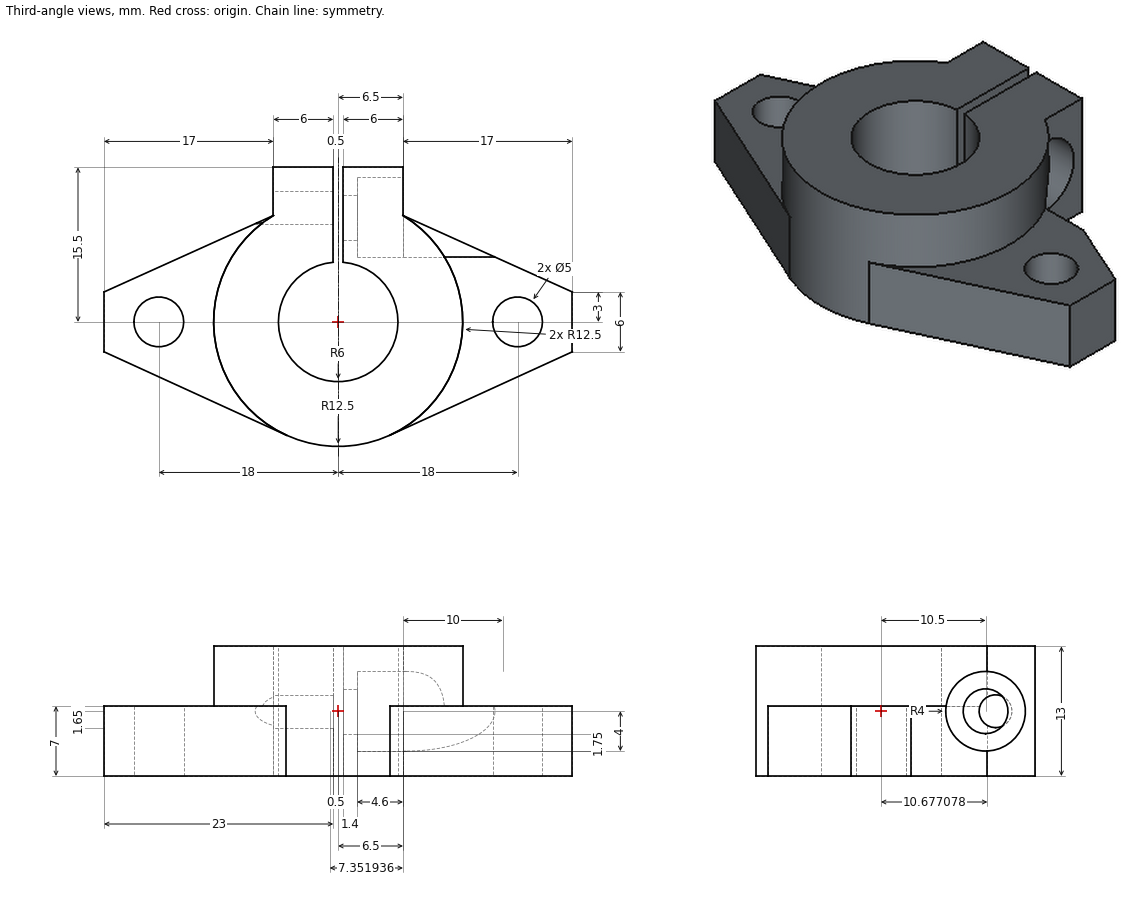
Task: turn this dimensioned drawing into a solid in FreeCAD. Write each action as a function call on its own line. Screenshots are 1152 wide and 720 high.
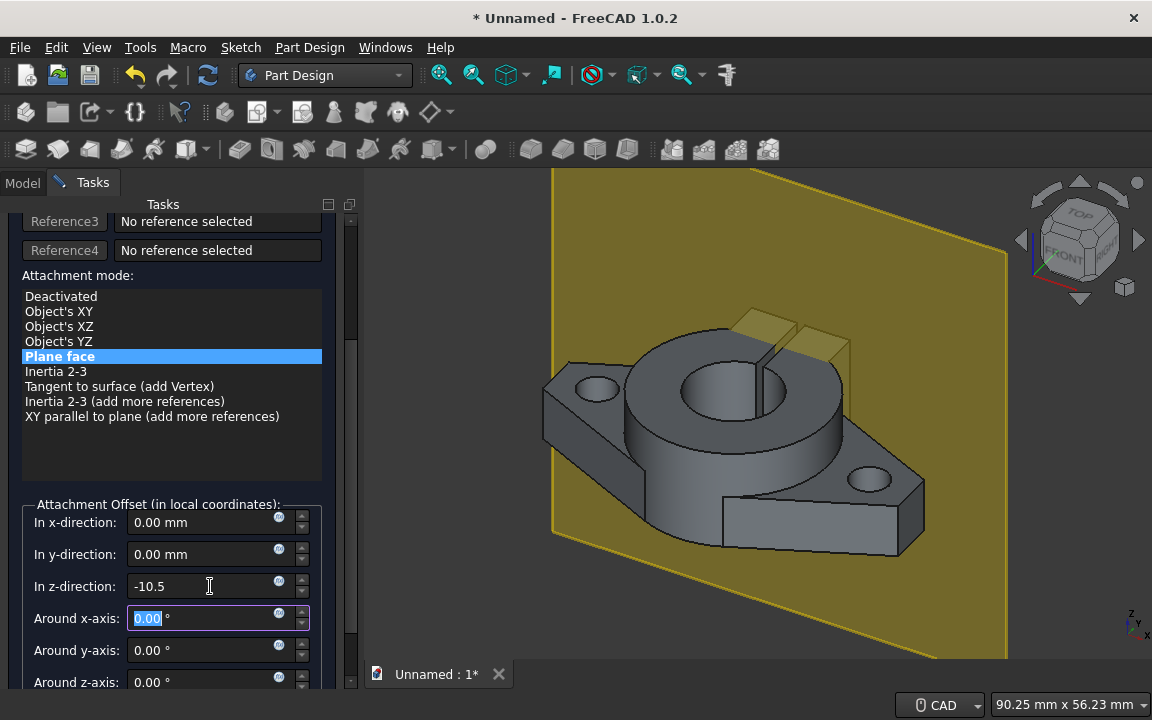
scroll(351, 451, up, 4)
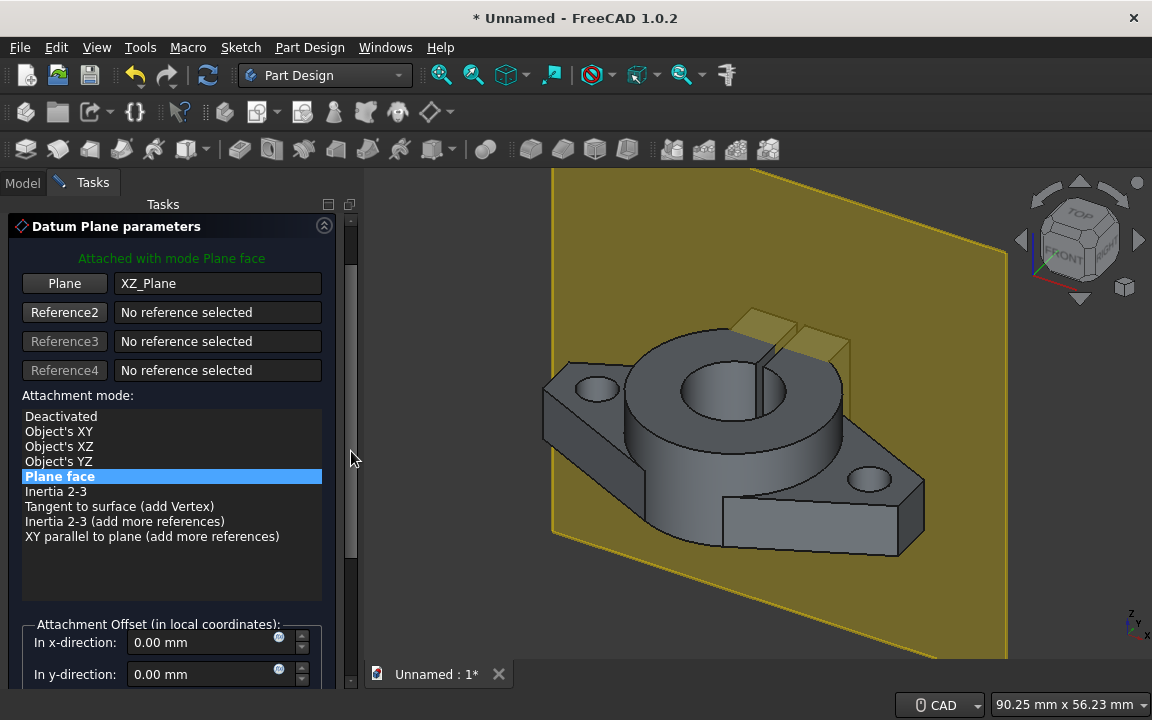
click(124, 243)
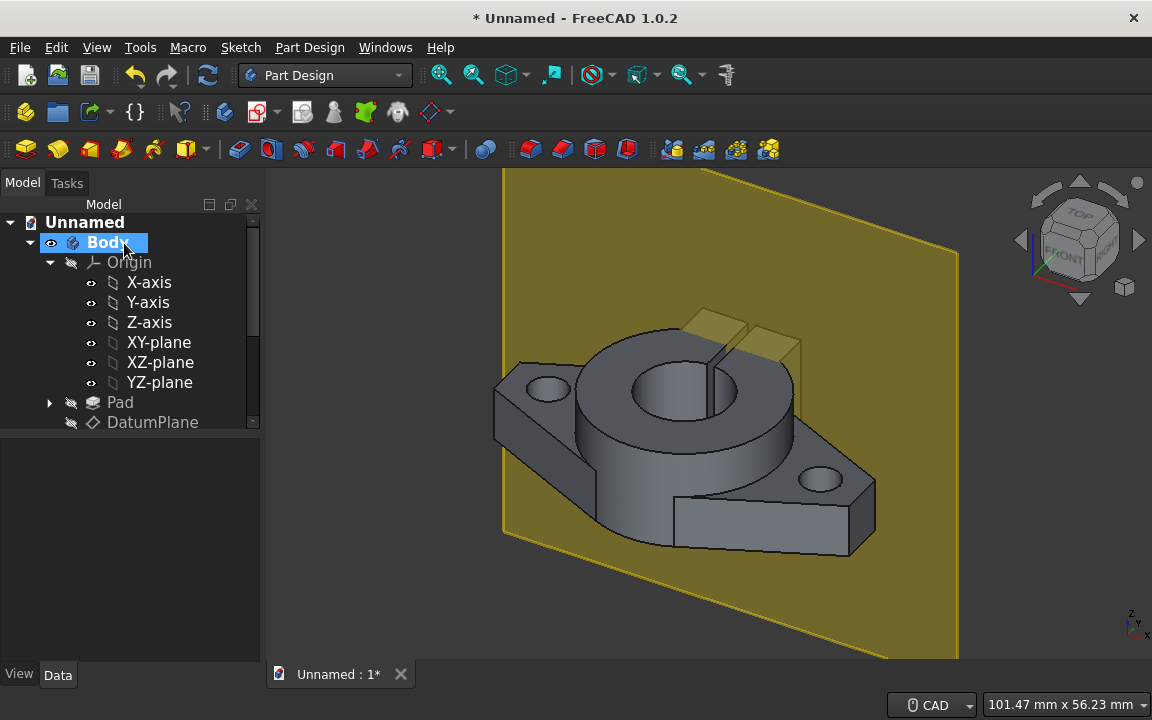
scroll(100, 318, down, 3)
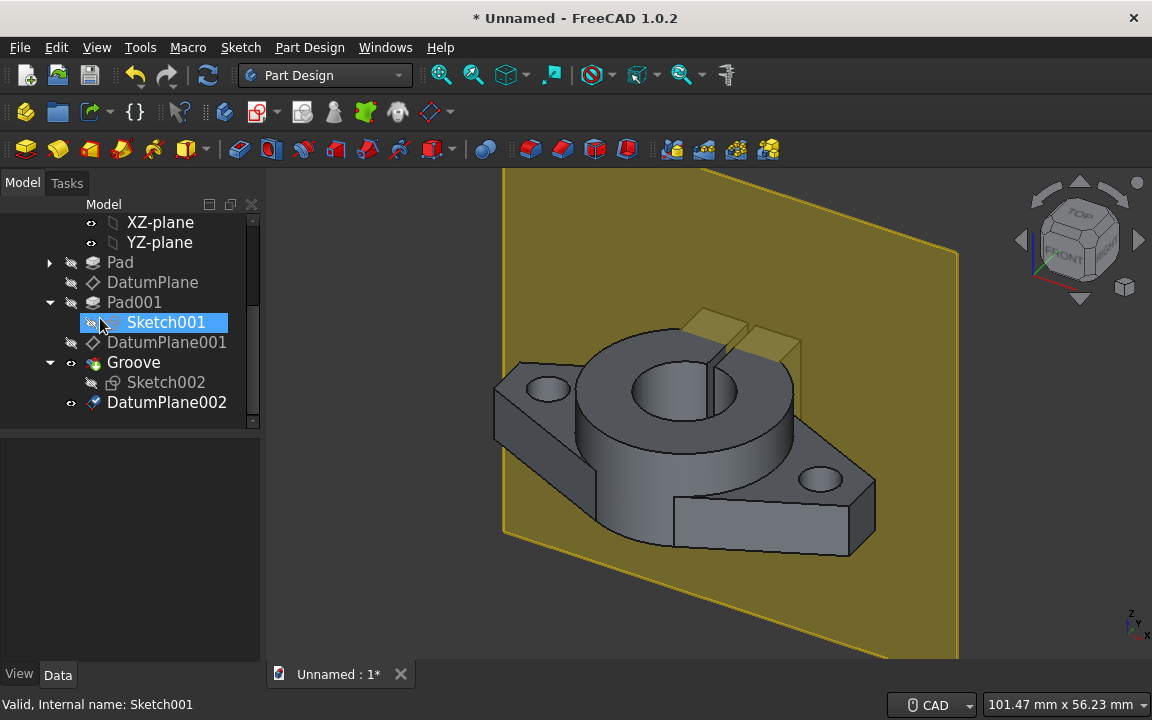
click(116, 403)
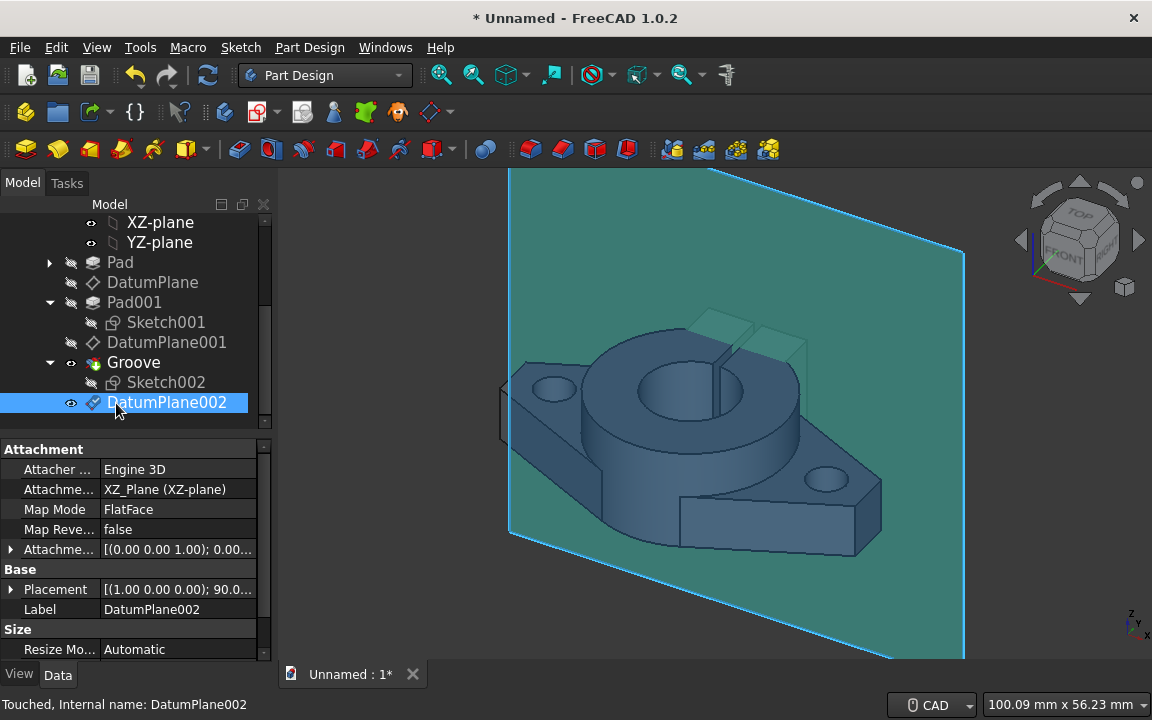
click(258, 112)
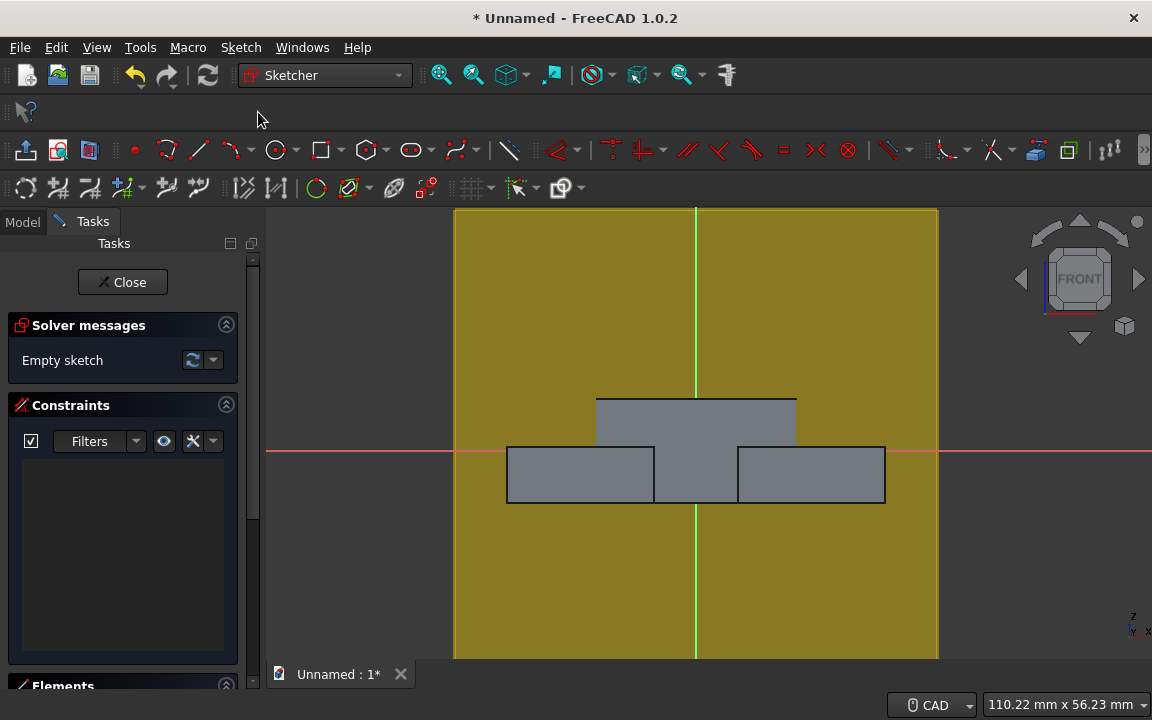
click(90, 150)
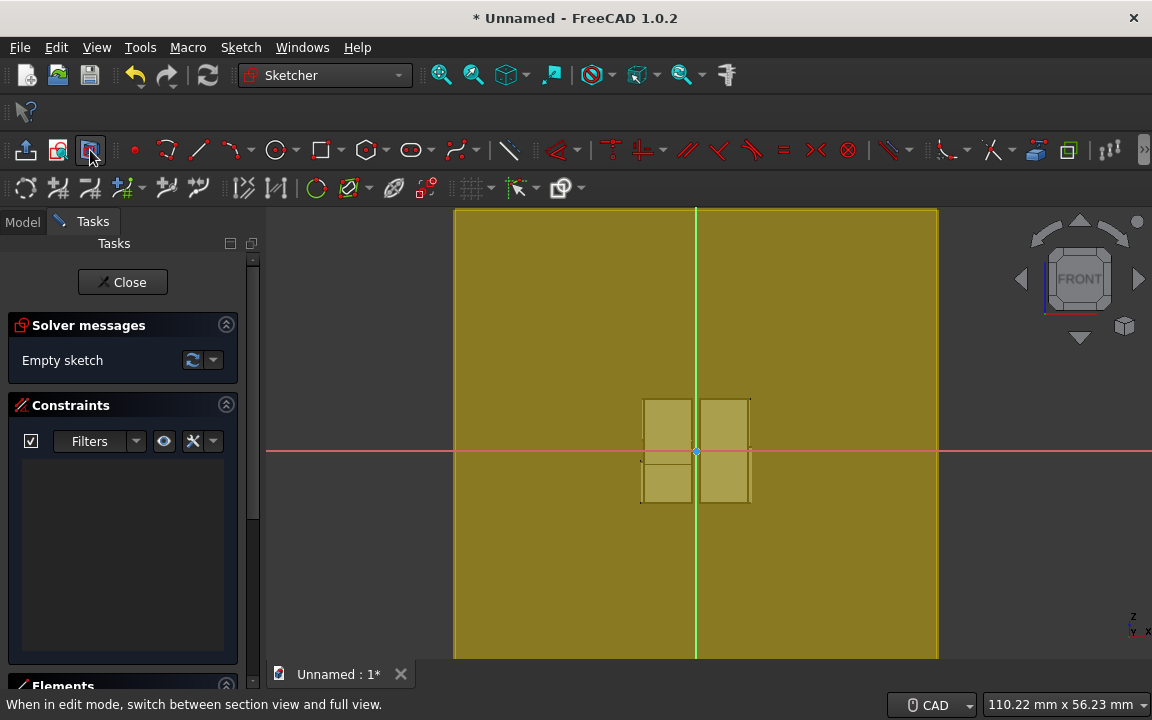
scroll(729, 471, up, 11)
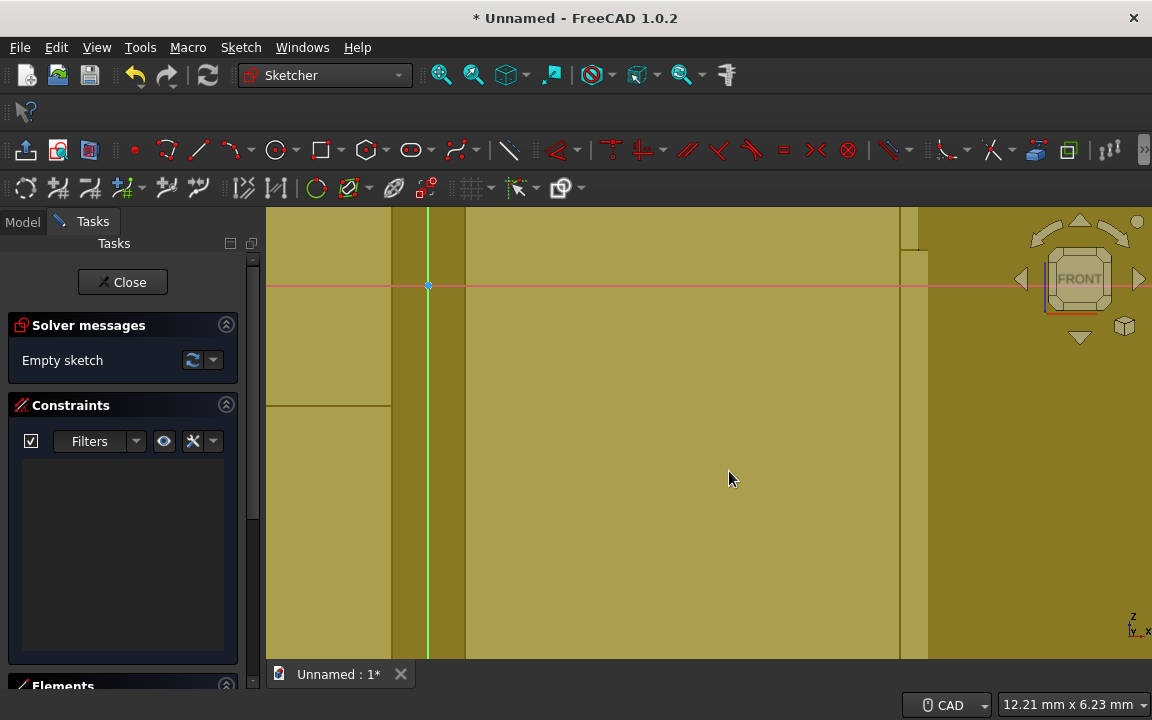
click(168, 150)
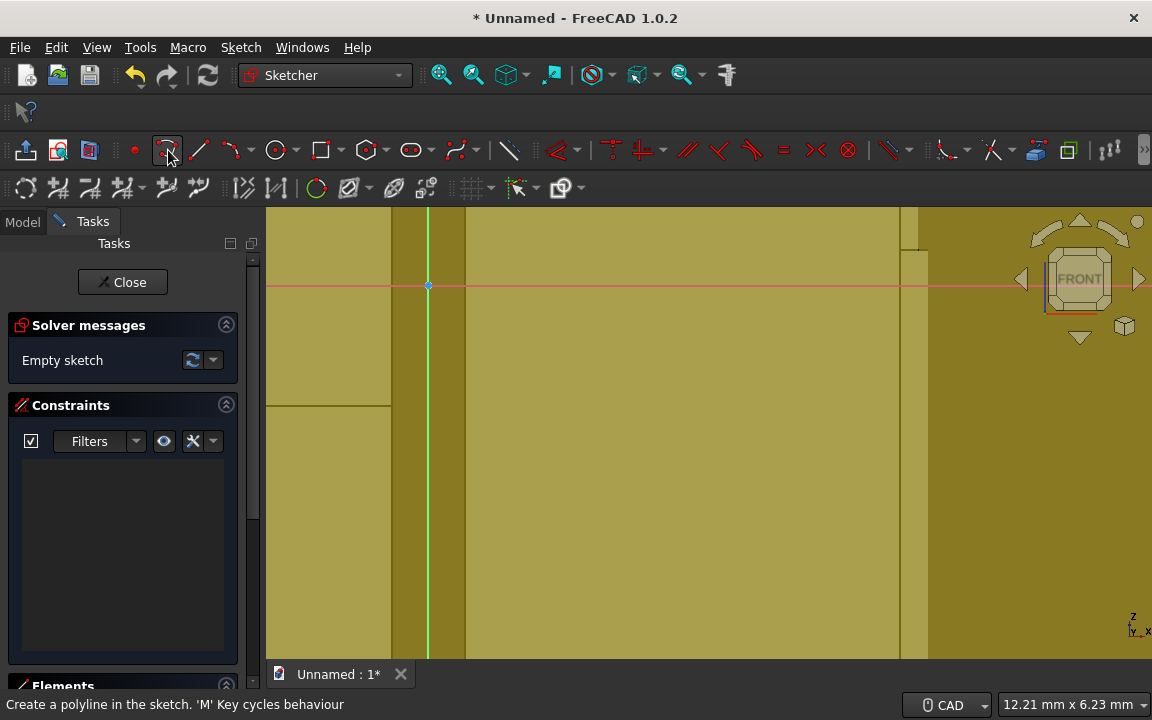
click(366, 286)
click(900, 295)
click(900, 576)
click(566, 576)
click(566, 449)
click(465, 449)
click(366, 286)
key(Escape)
key(Escape)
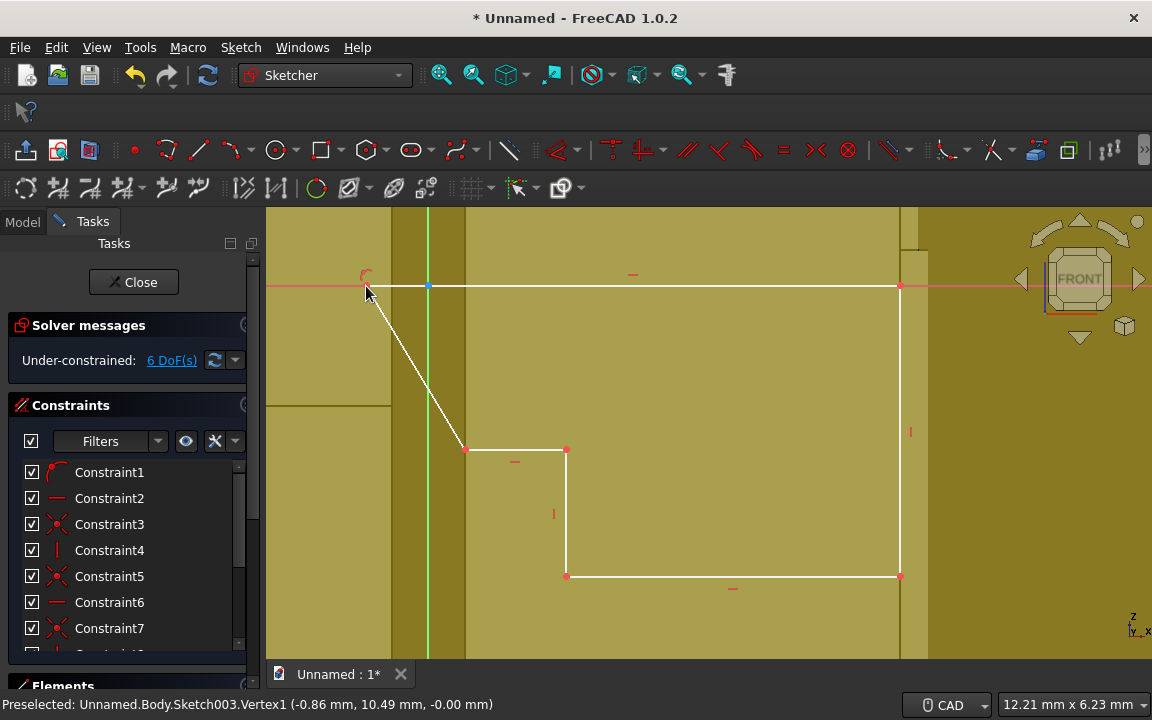
click(556, 150)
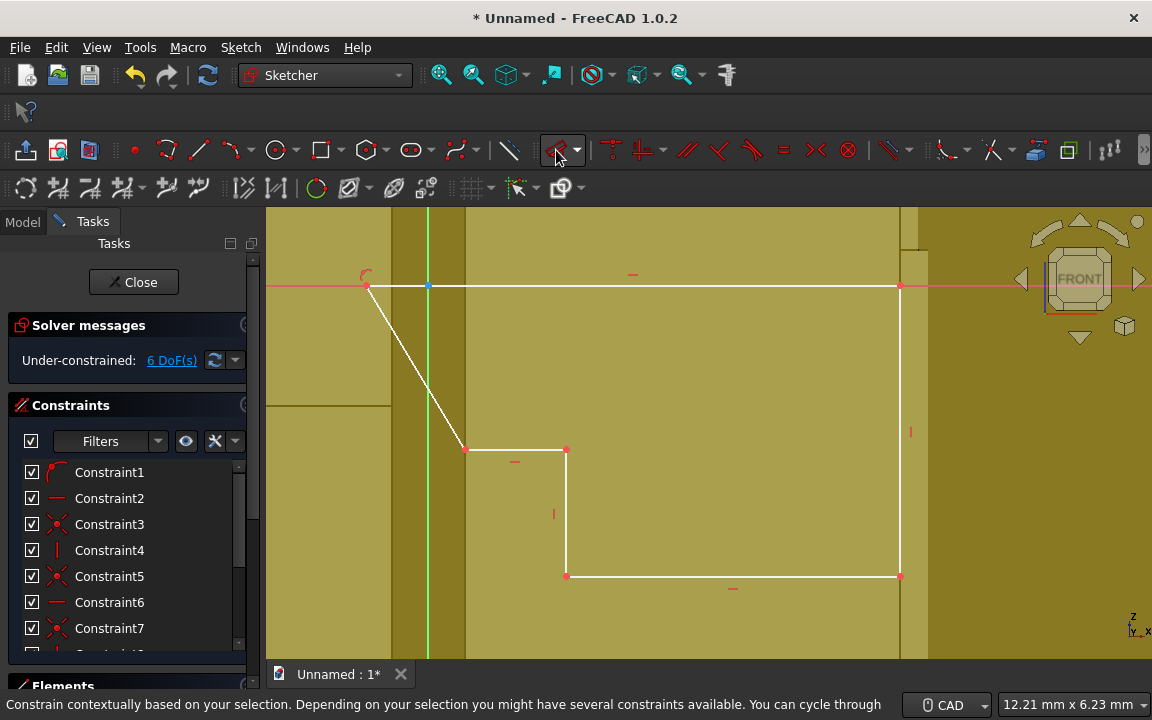
click(900, 373)
click(934, 431)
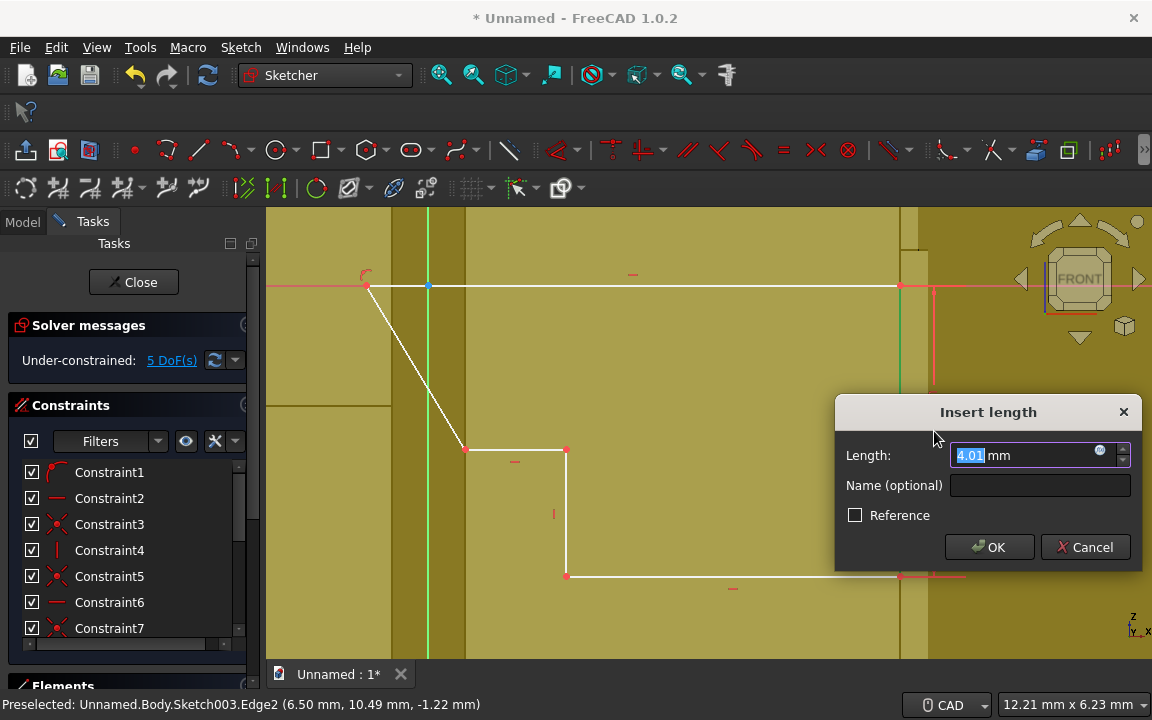
text(4)
key(Return)